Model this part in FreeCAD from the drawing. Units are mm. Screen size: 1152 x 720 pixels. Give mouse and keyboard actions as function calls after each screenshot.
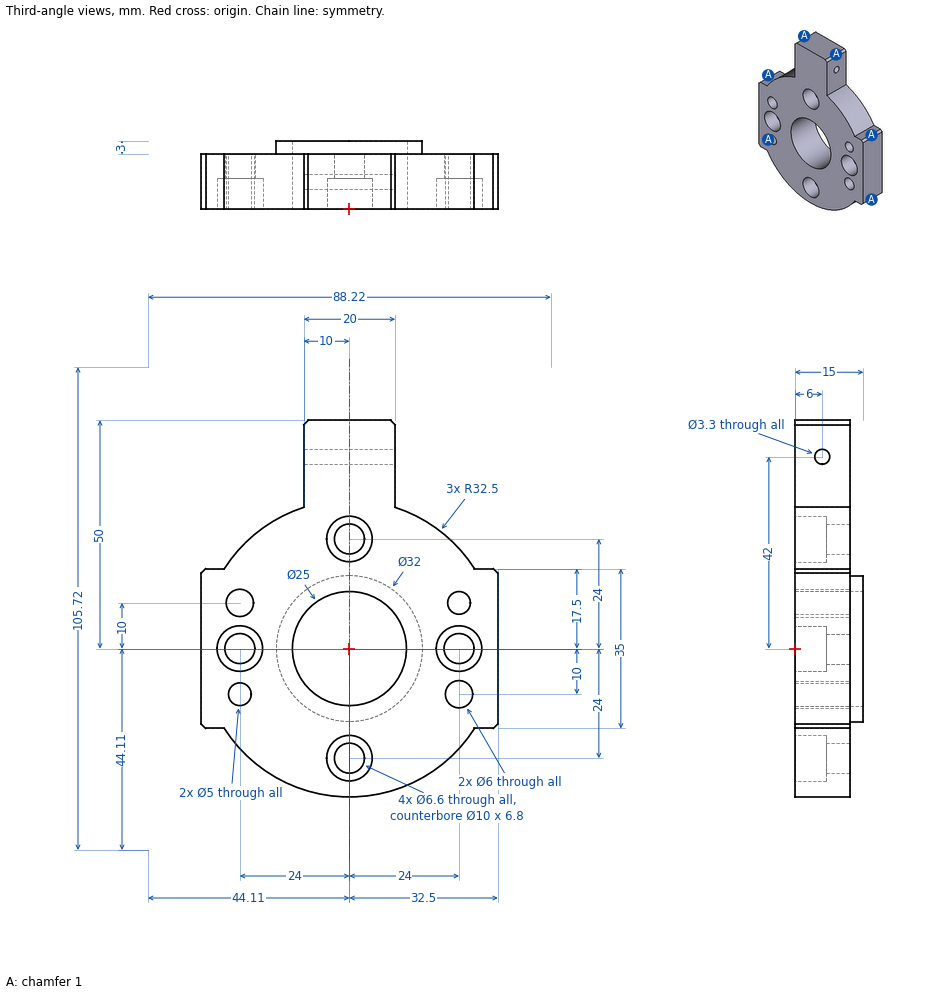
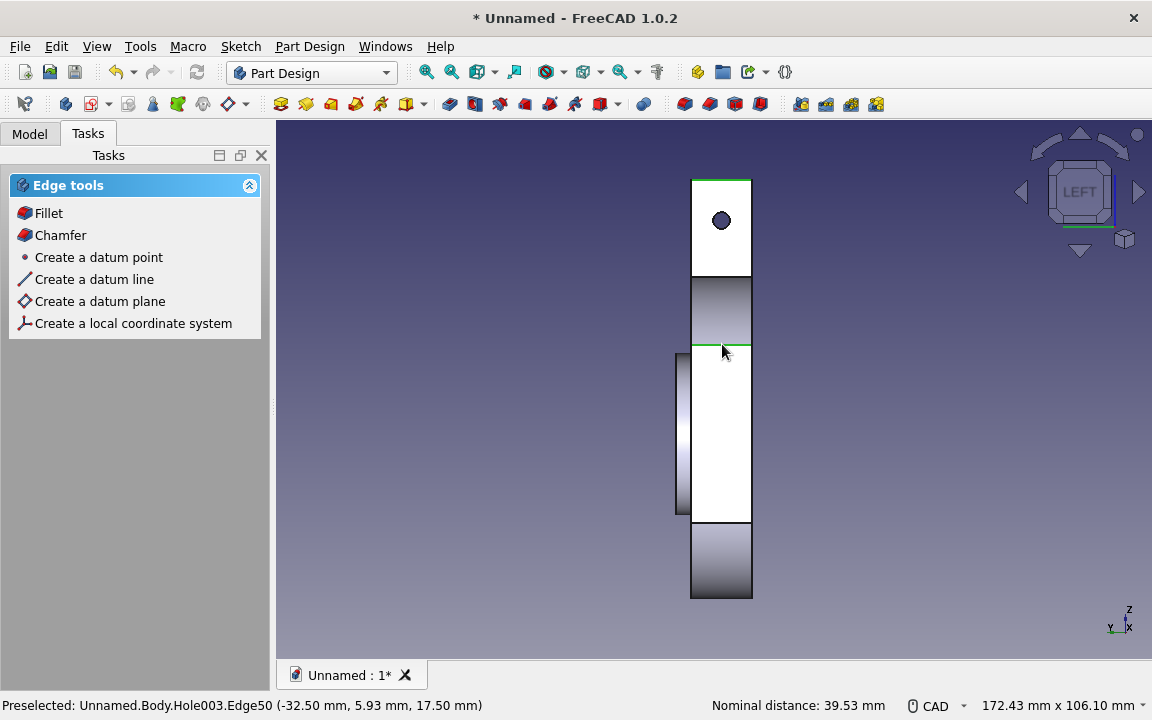
click(722, 522, ctrl)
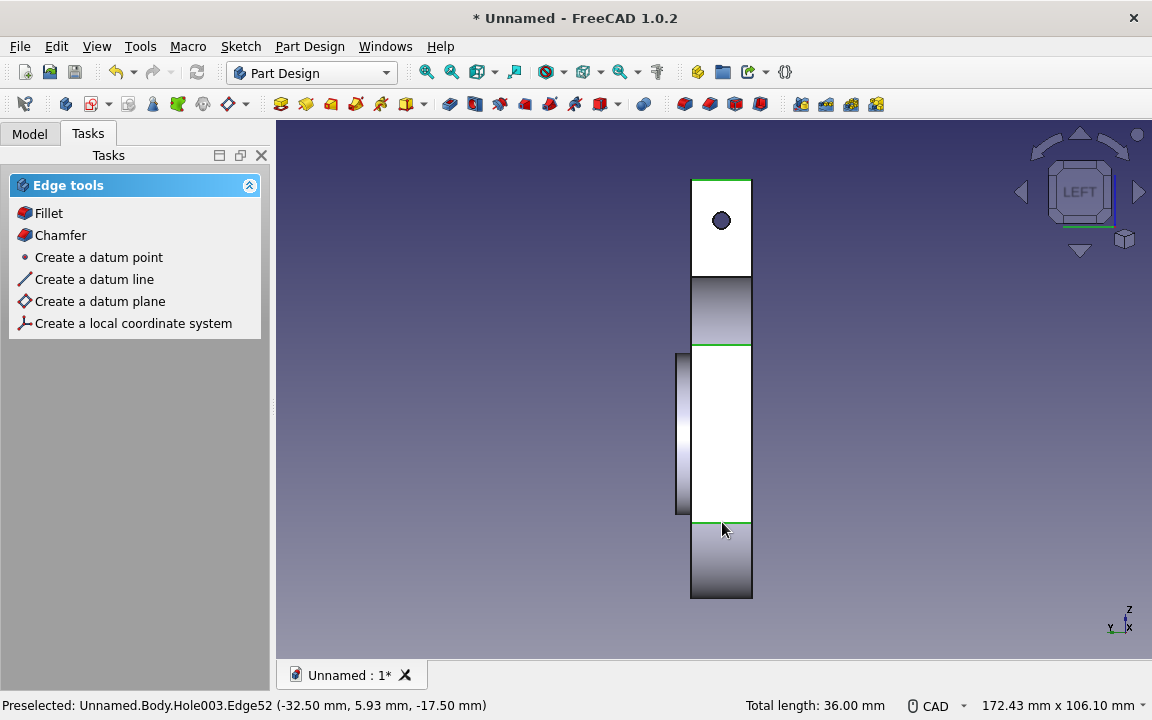
key(0)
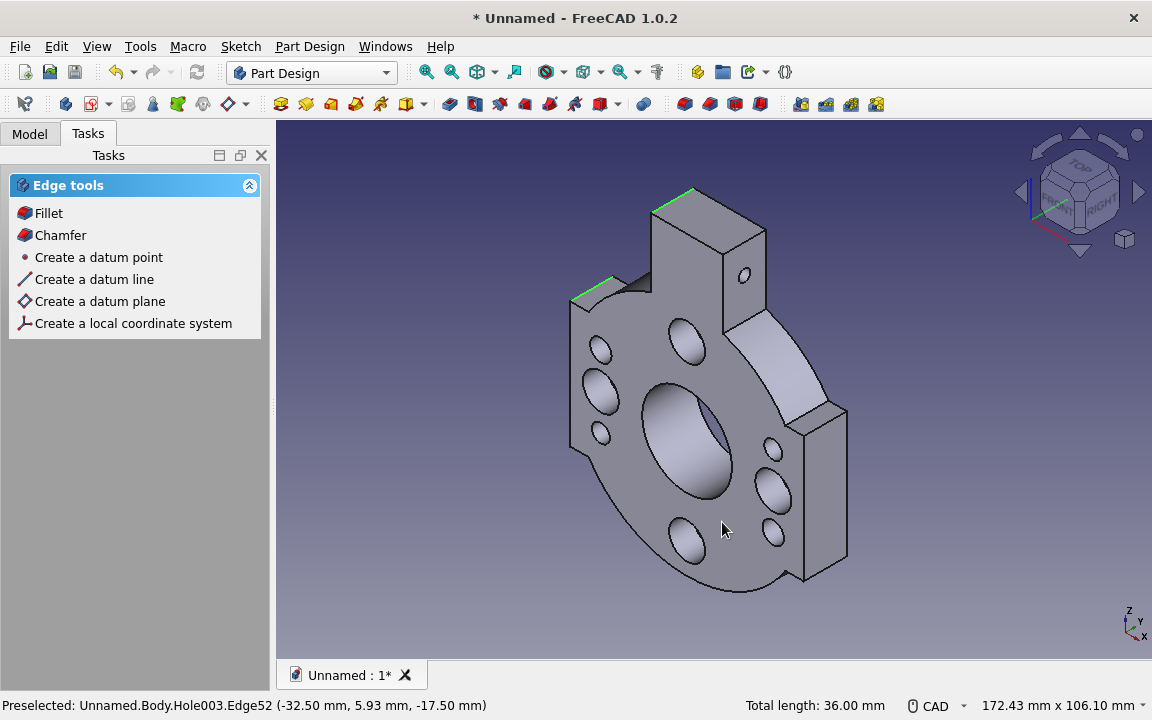
click(745, 241, ctrl)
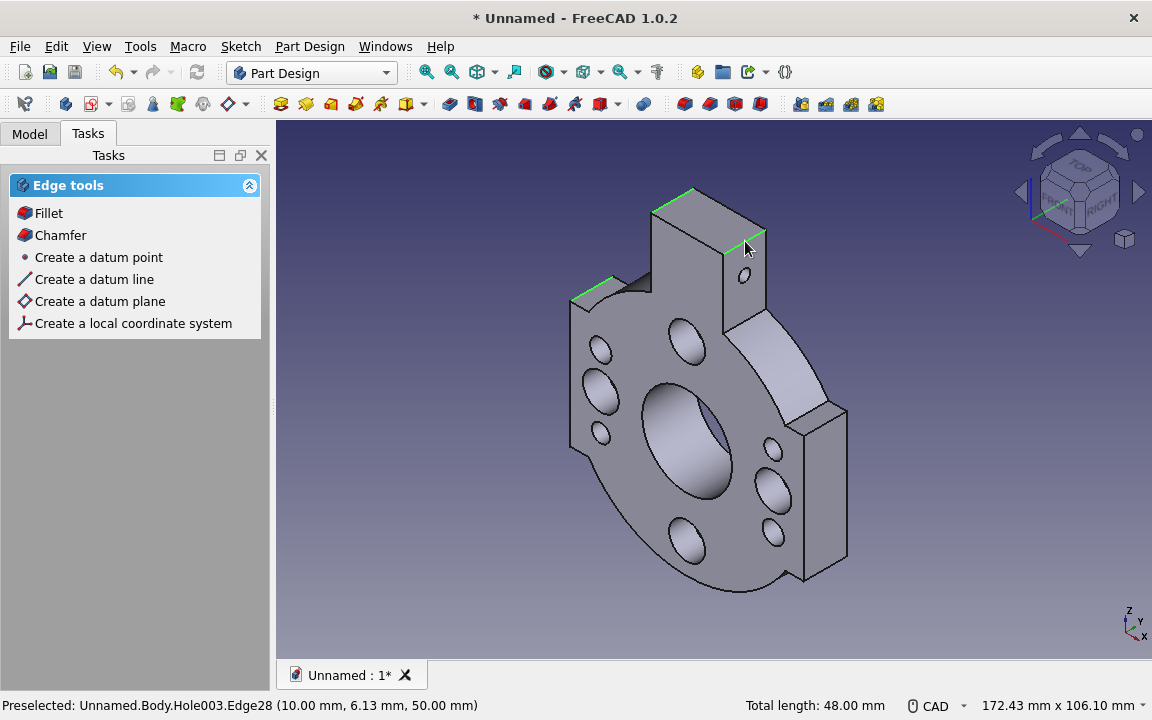
click(825, 423, ctrl)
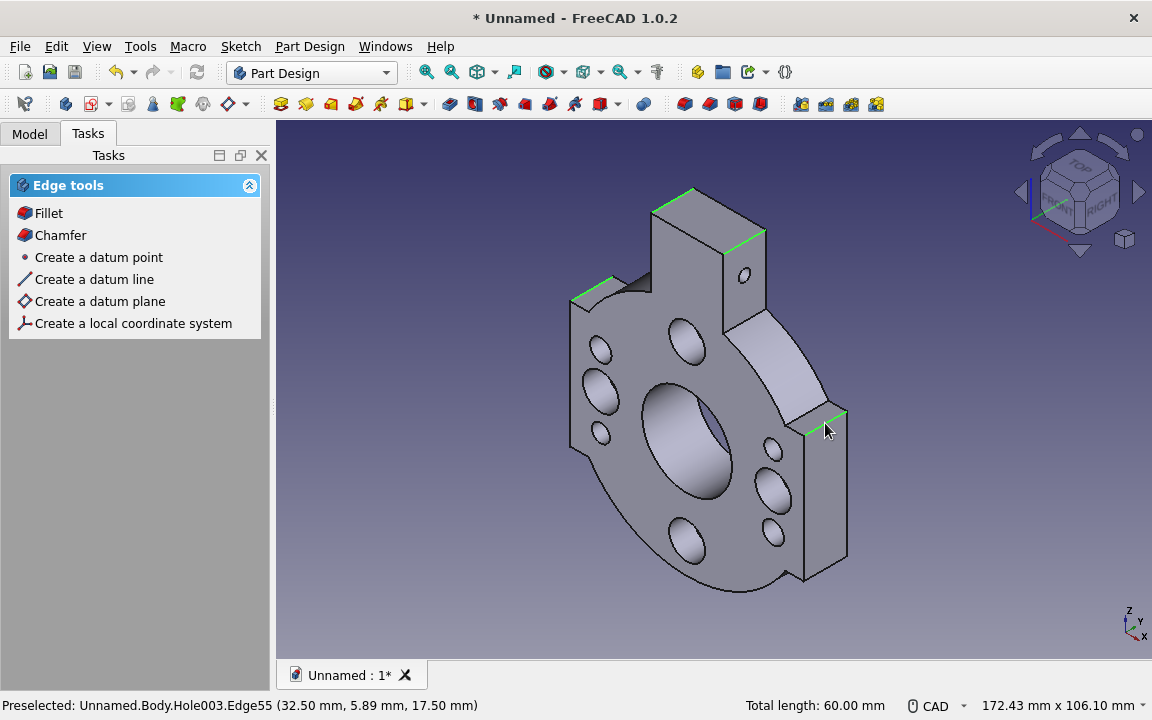
key(2)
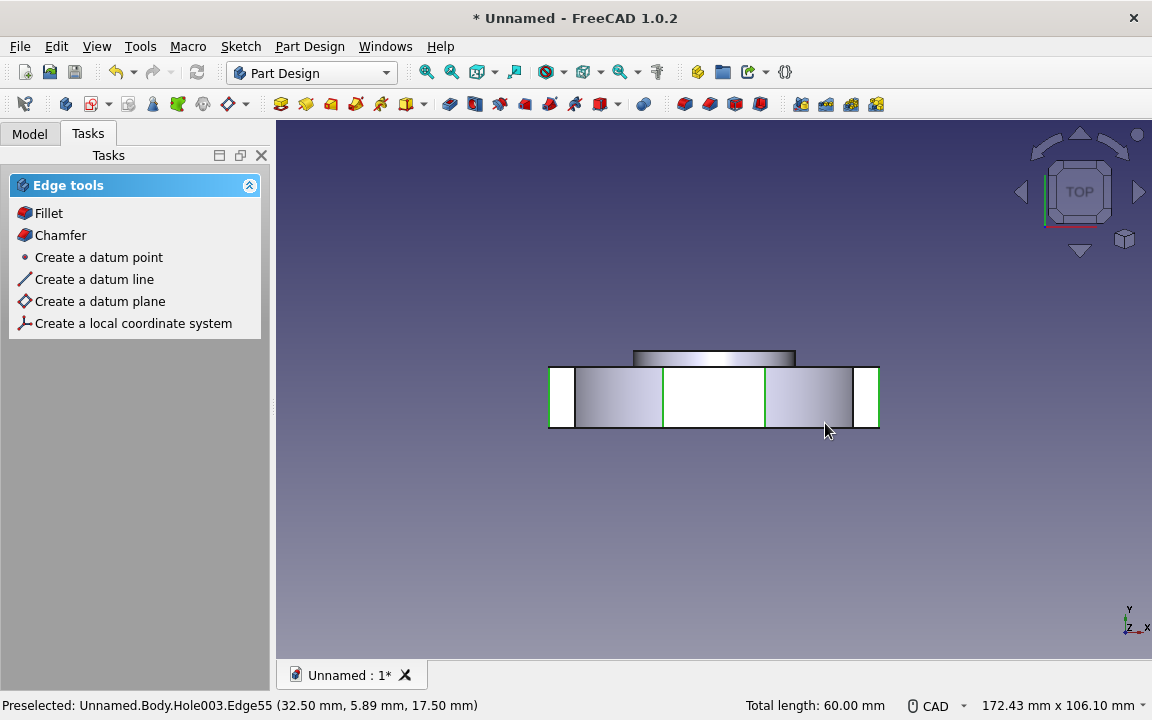
key(v)
key(f)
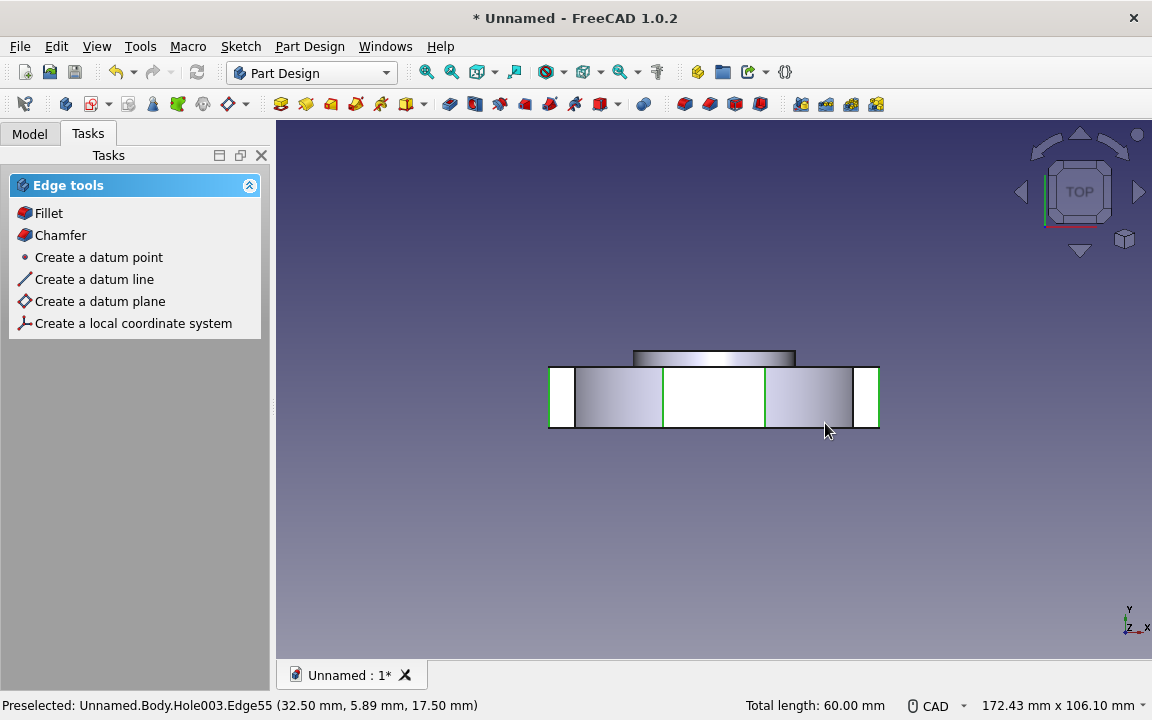
key(1)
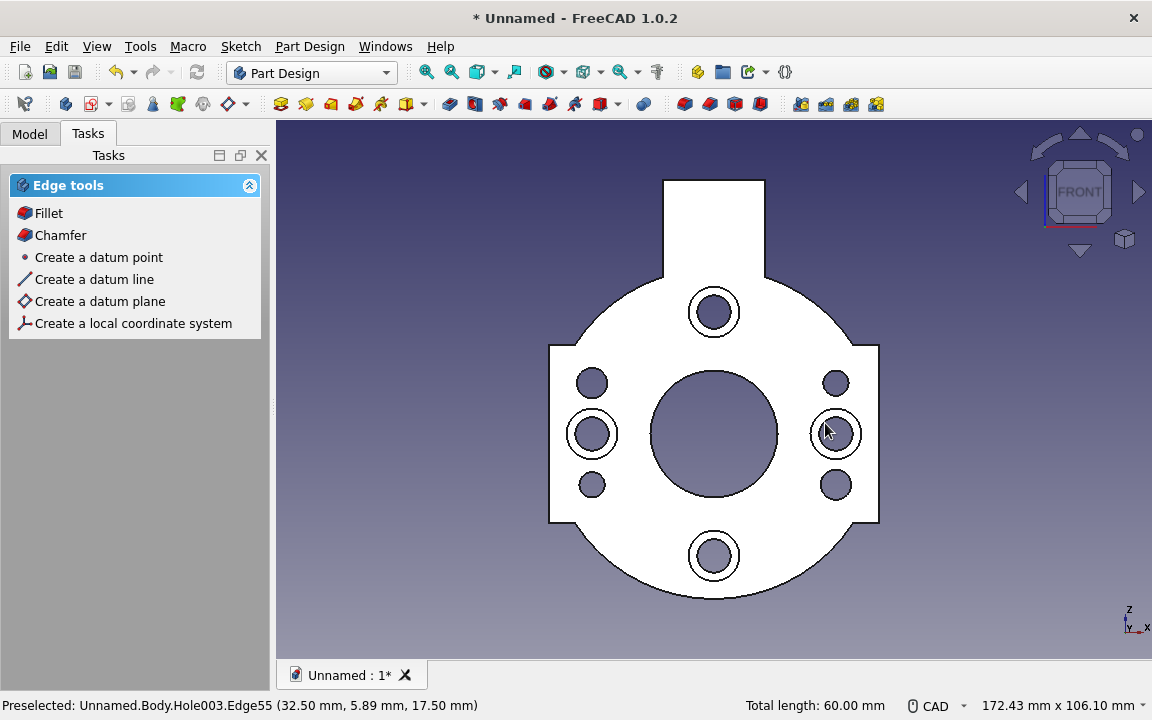
key(3)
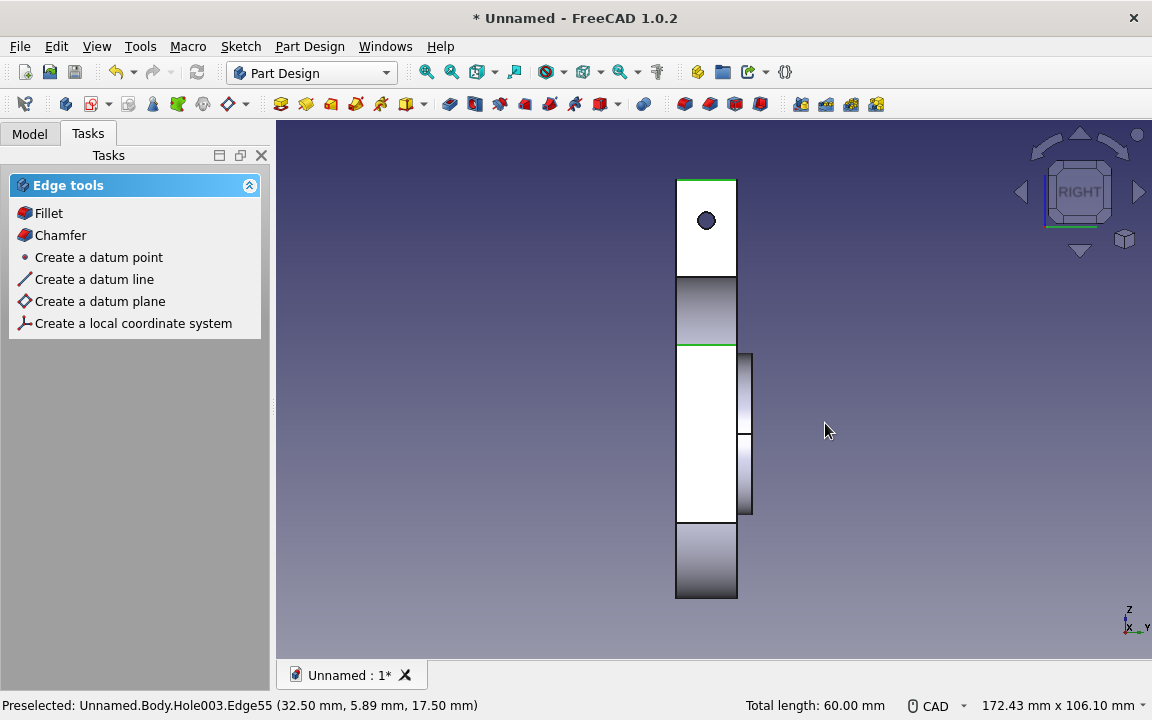
click(706, 522, ctrl)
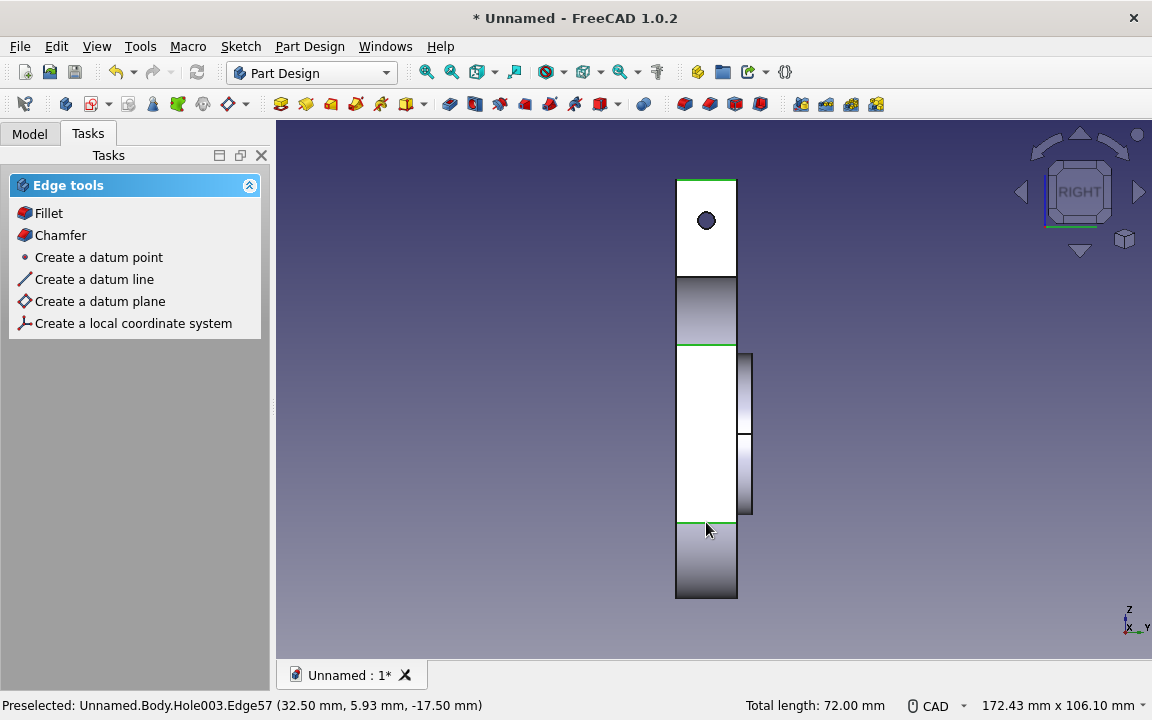
click(710, 104)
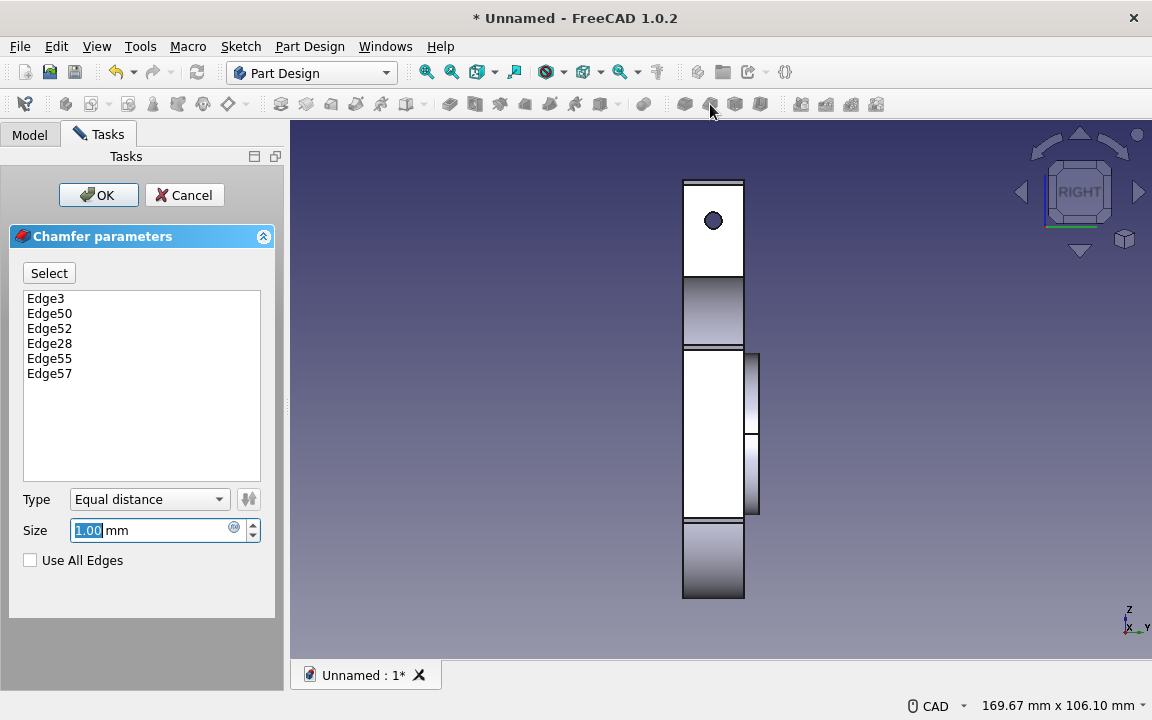
text(1)
key(Tab)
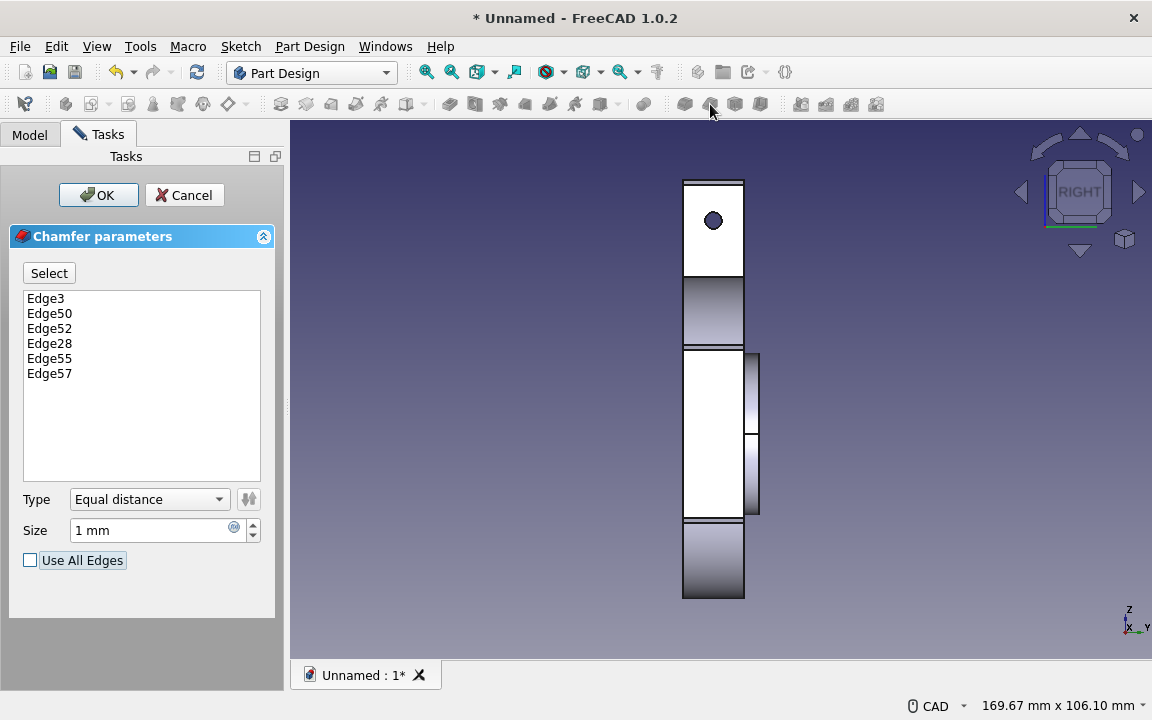
click(99, 195)